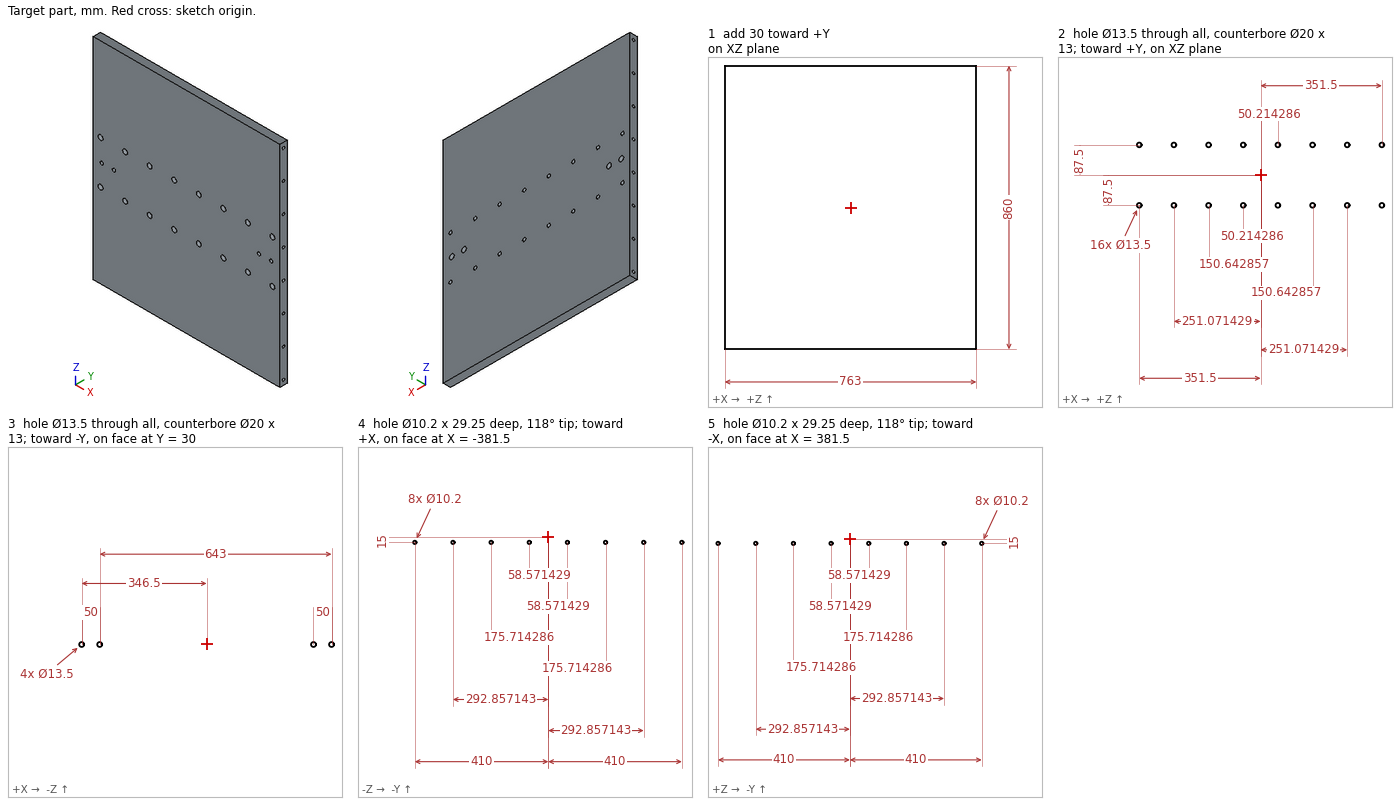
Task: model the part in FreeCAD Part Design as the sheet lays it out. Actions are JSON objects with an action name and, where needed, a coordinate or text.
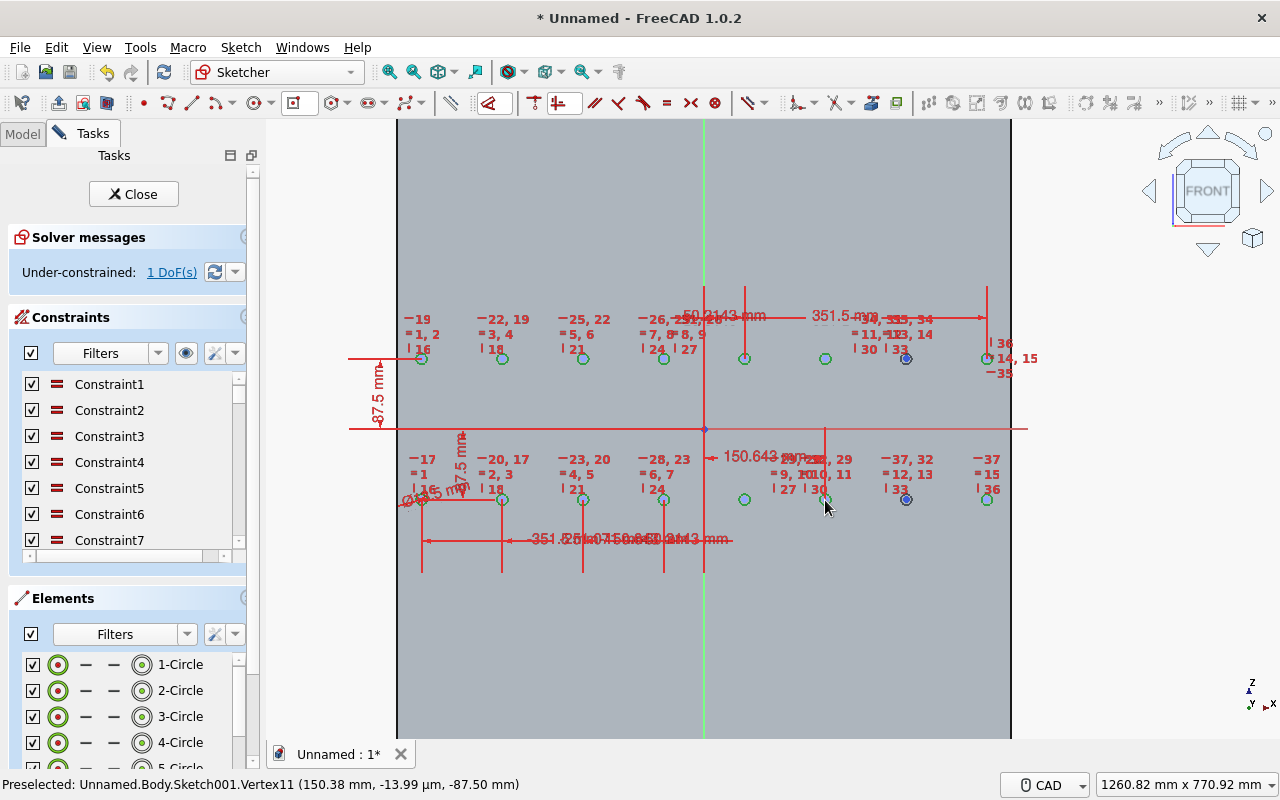
{"action": "left_click", "coordinate": [906, 500]}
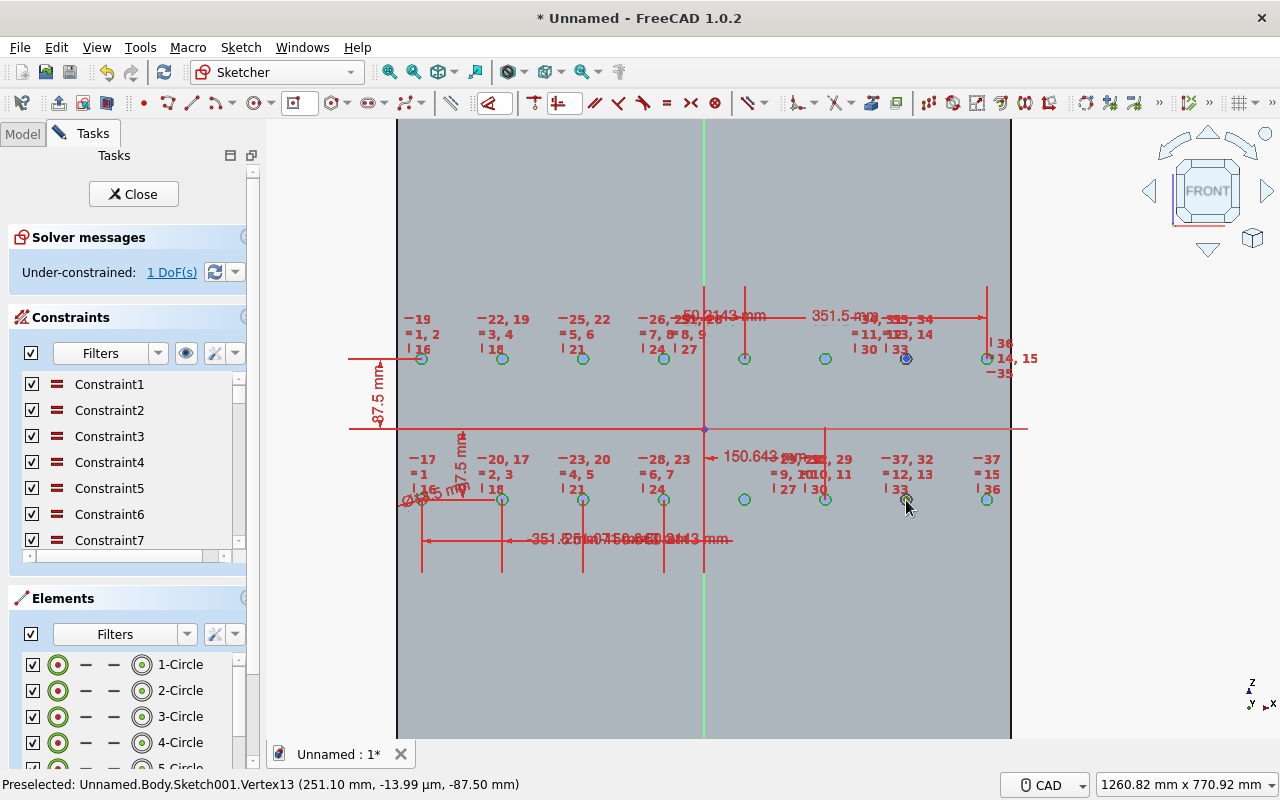
{"action": "left_click", "coordinate": [506, 104]}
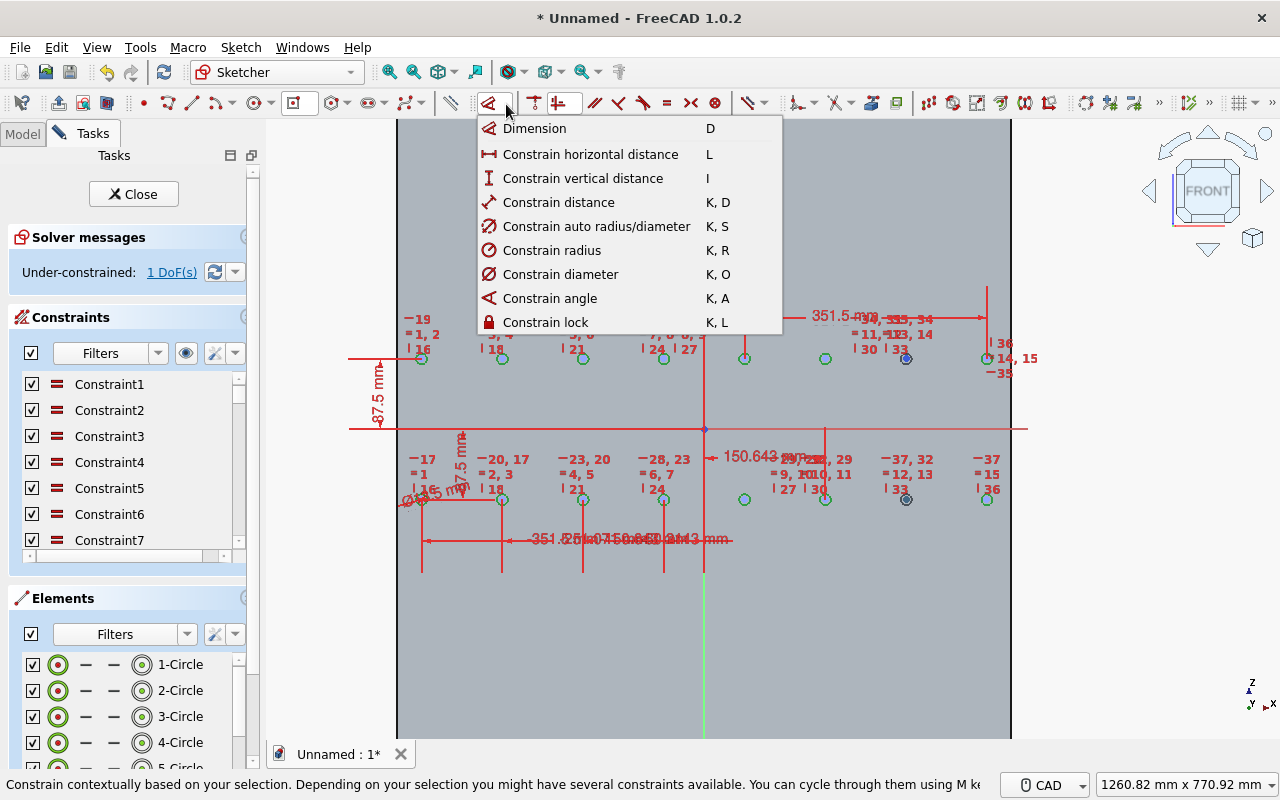
{"action": "left_click", "coordinate": [630, 154]}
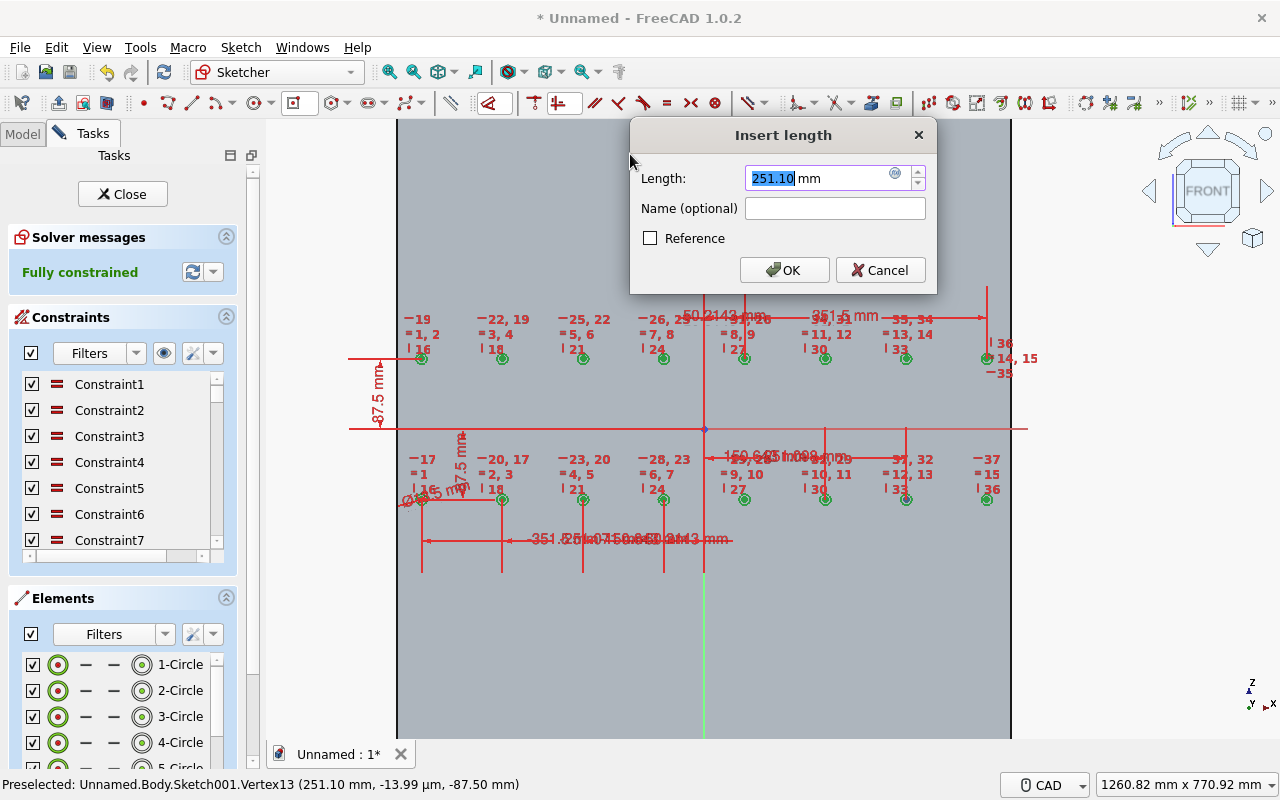
{"action": "type", "text": "251.071429"}
{"action": "key", "text": "Return"}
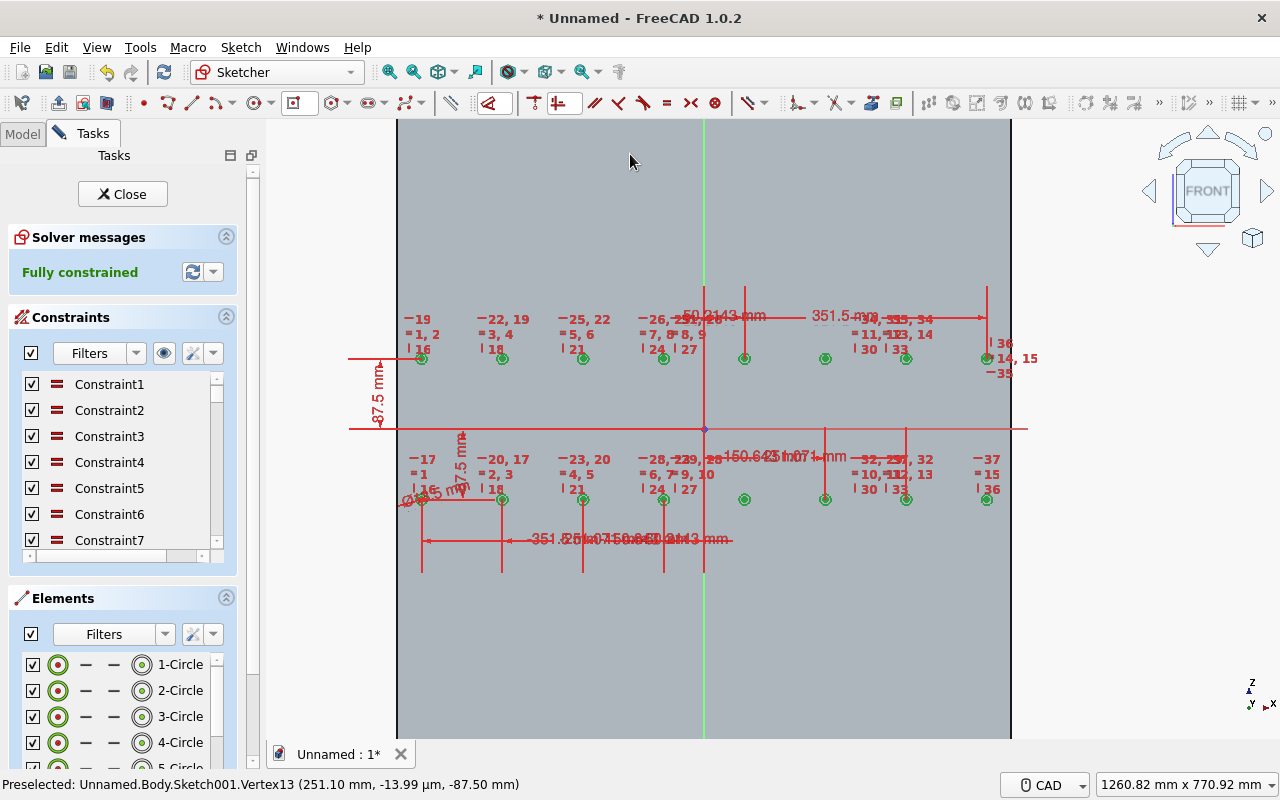
{"action": "left_click", "coordinate": [123, 194]}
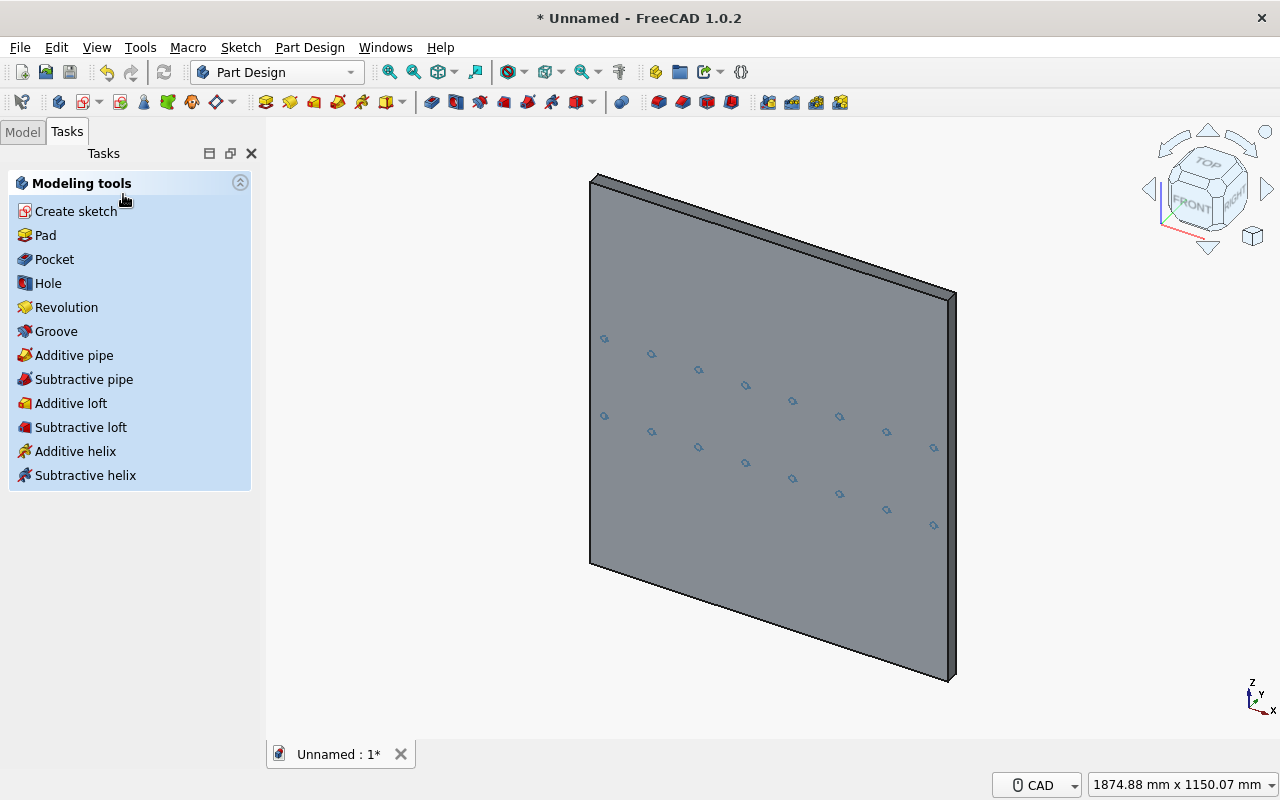
{"action": "left_click", "coordinate": [456, 102]}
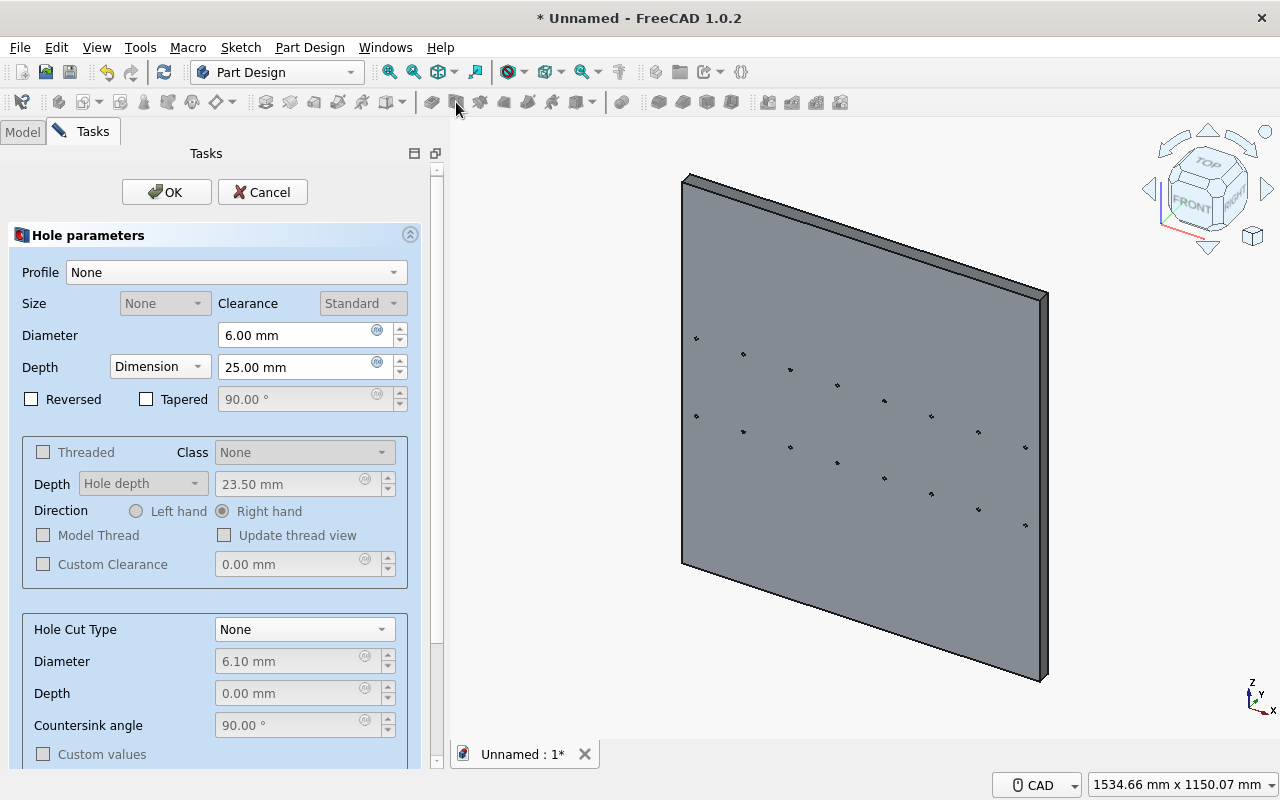
{"action": "triple_click", "coordinate": [305, 335]}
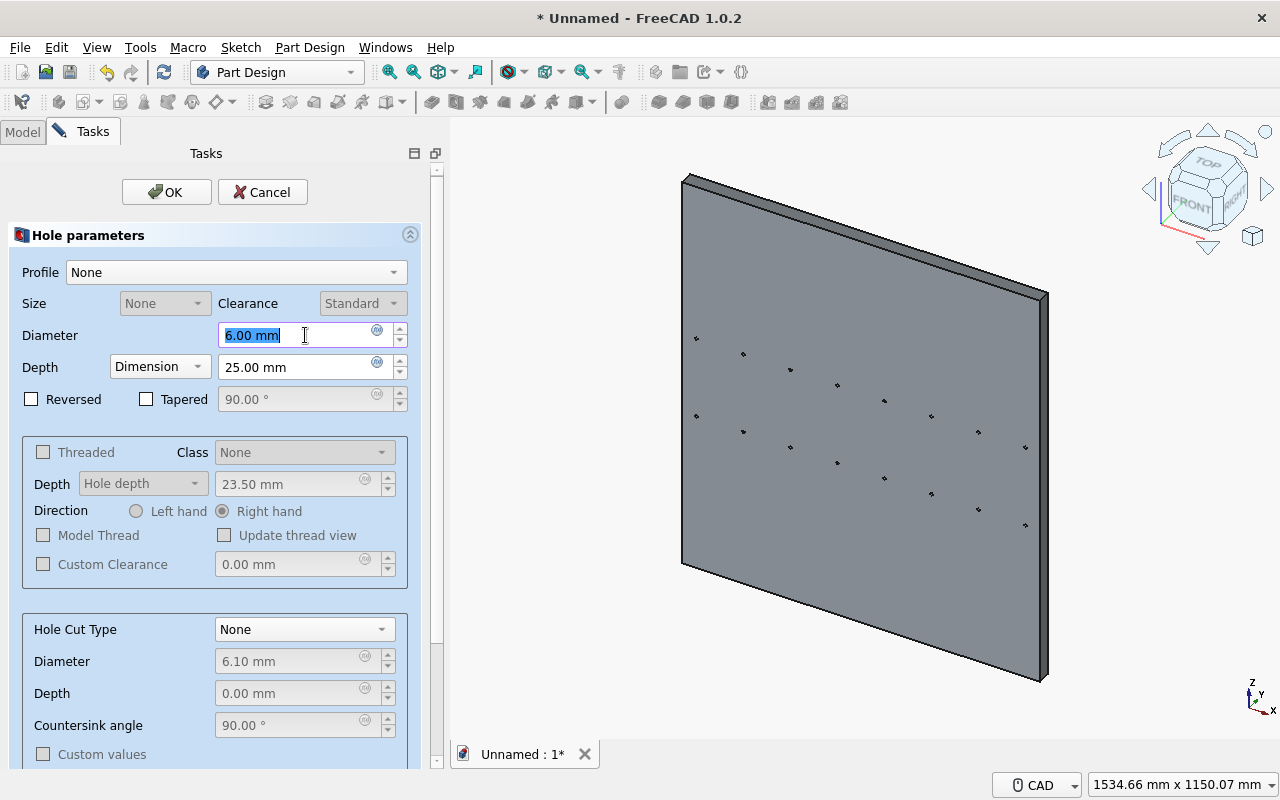
{"action": "type", "text": "13.5"}
{"action": "key", "text": "Tab"}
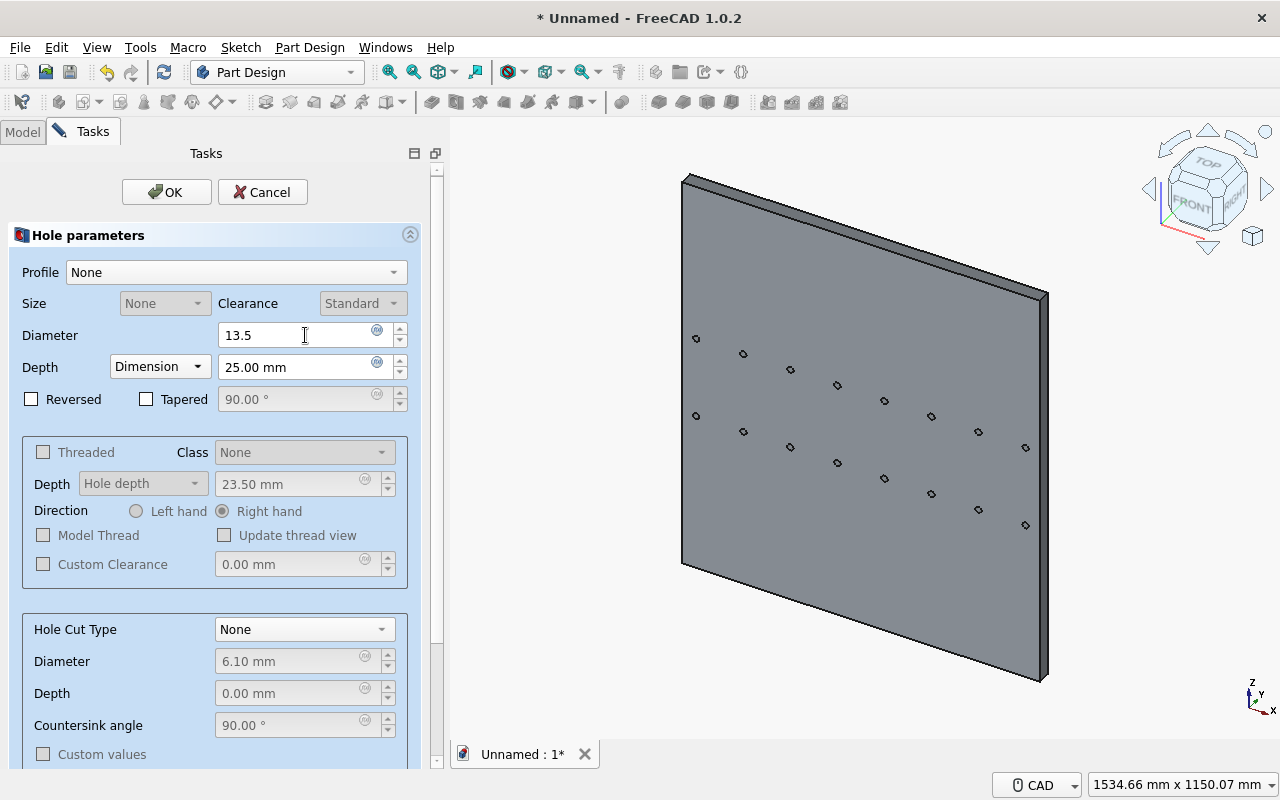
{"action": "left_click", "coordinate": [161, 366]}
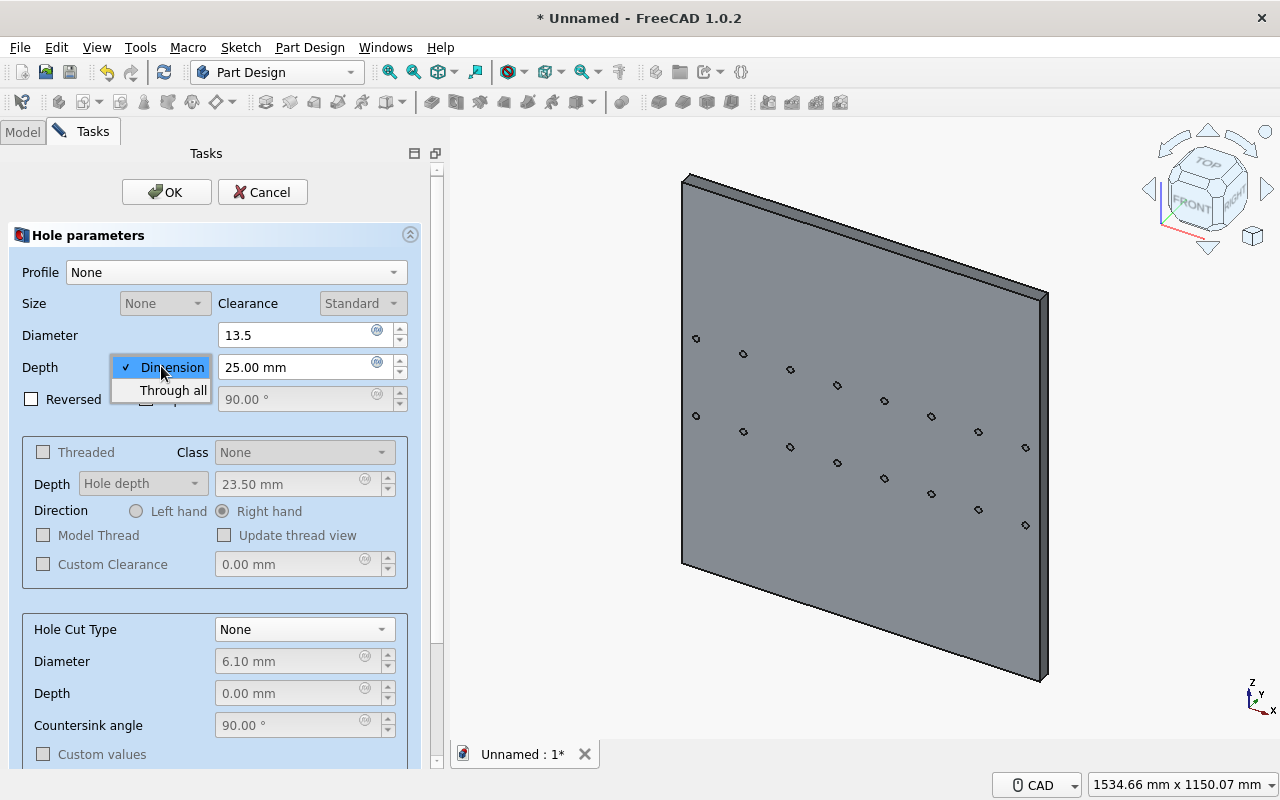
{"action": "left_click", "coordinate": [160, 390]}